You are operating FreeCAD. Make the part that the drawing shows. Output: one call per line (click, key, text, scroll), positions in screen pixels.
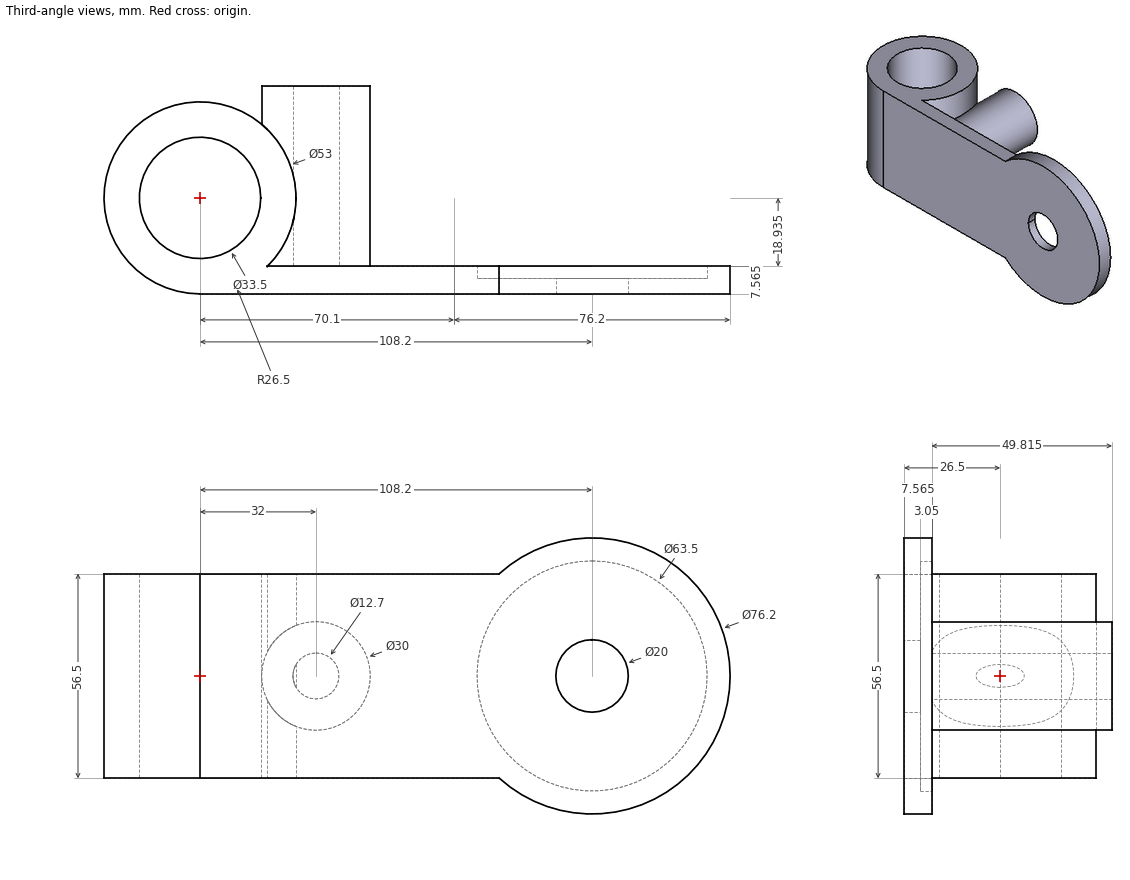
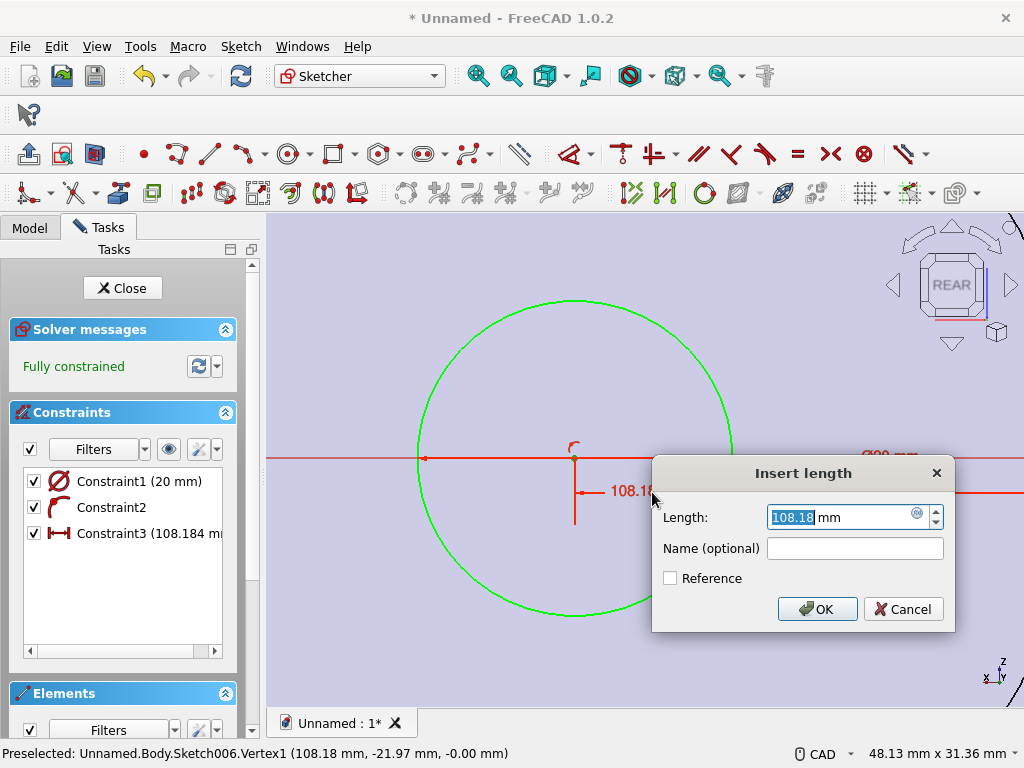
text(108.2)
key(Return)
key(Escape)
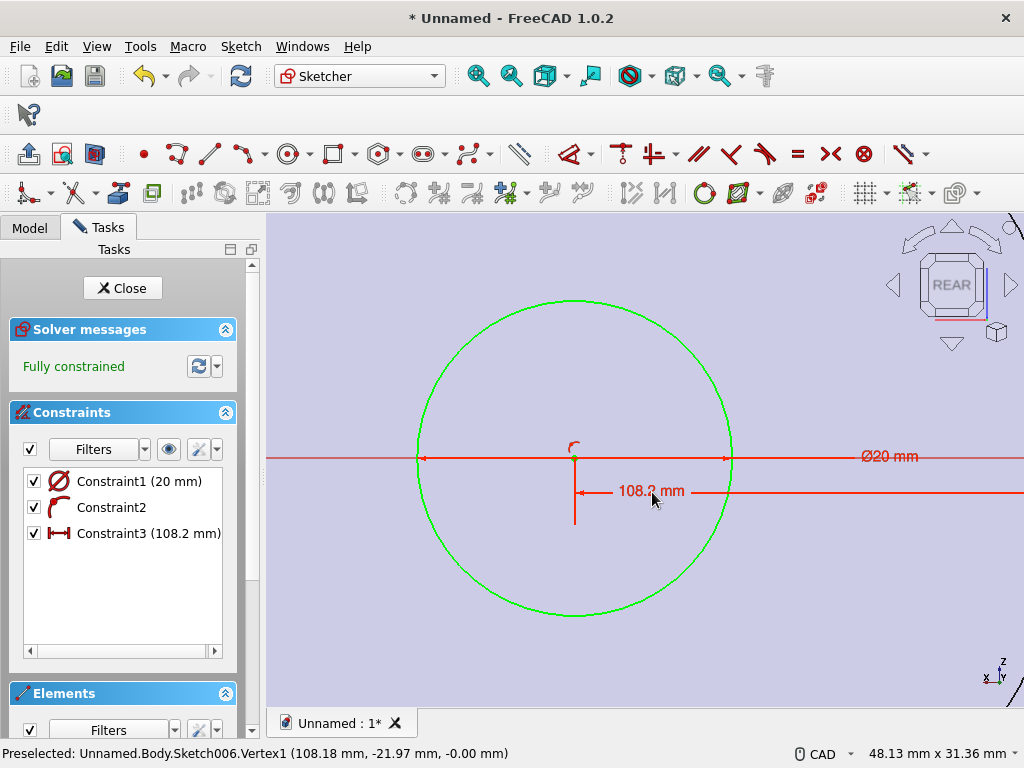
click(123, 288)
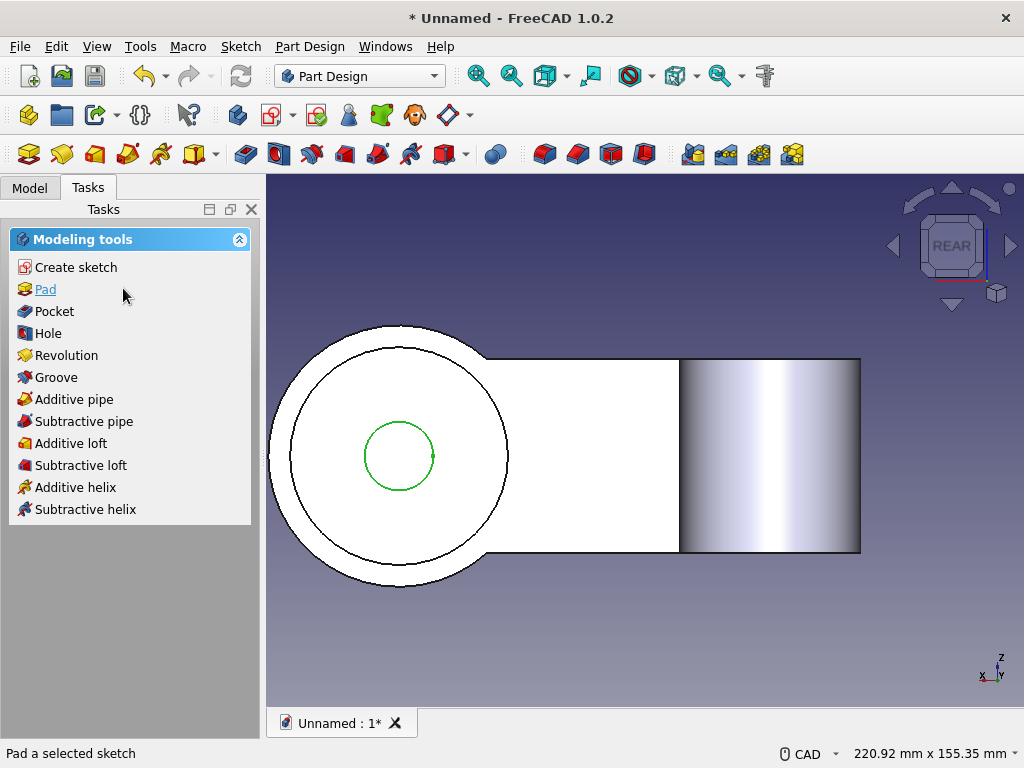
click(246, 154)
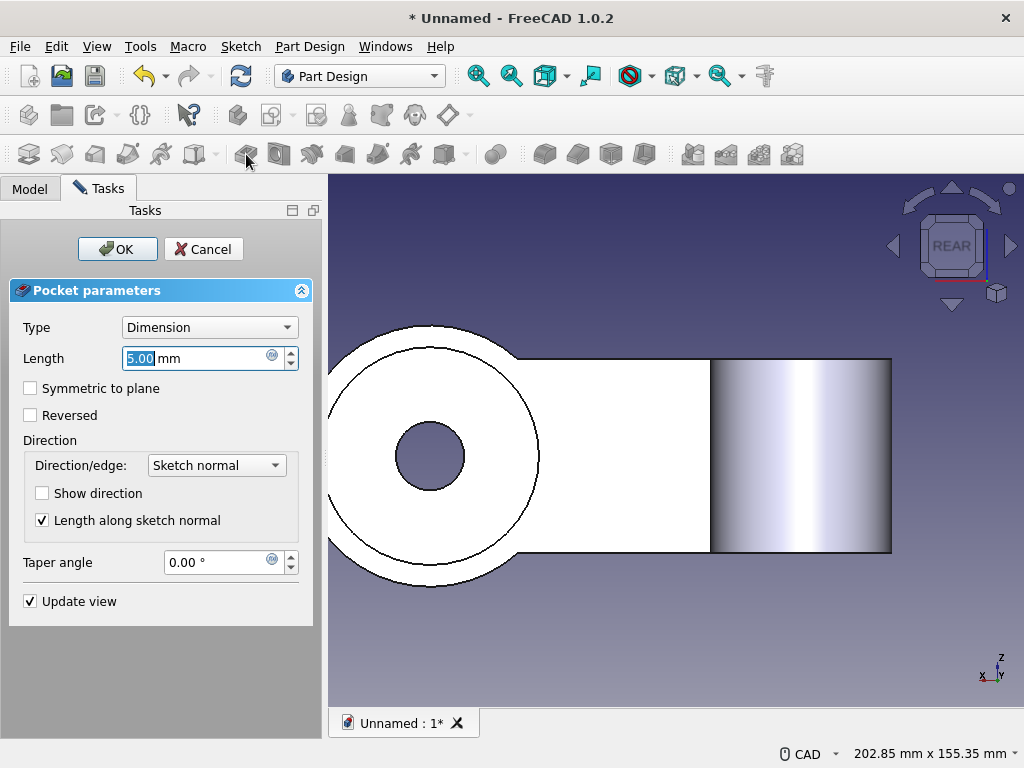
click(210, 328)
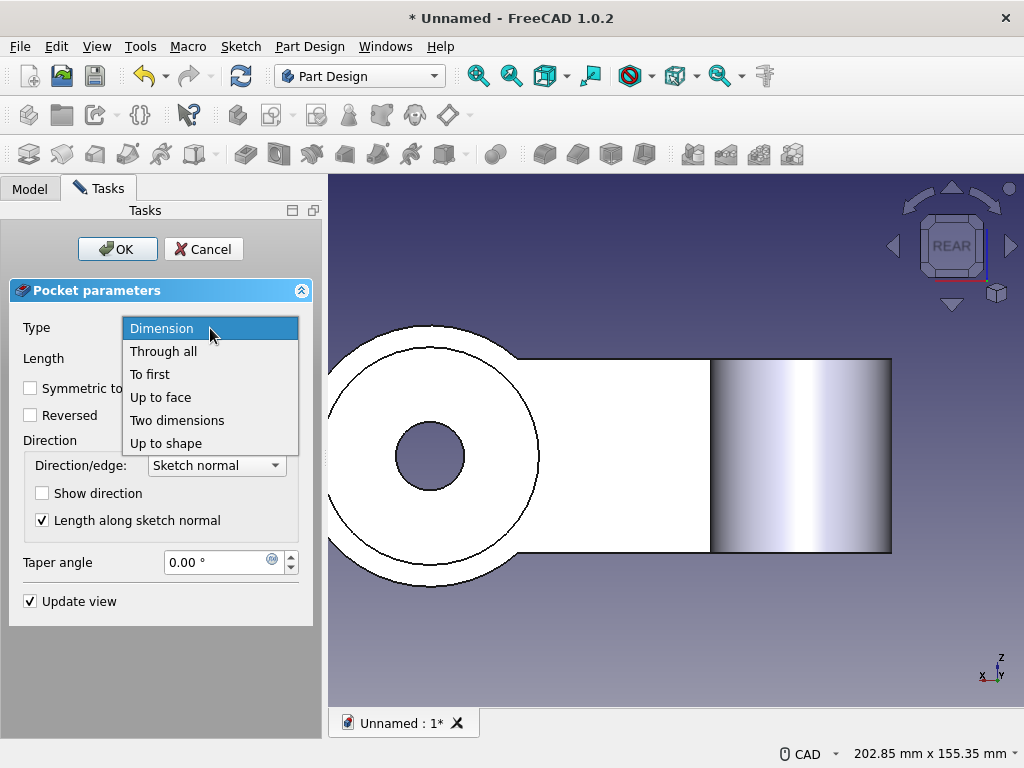
click(208, 352)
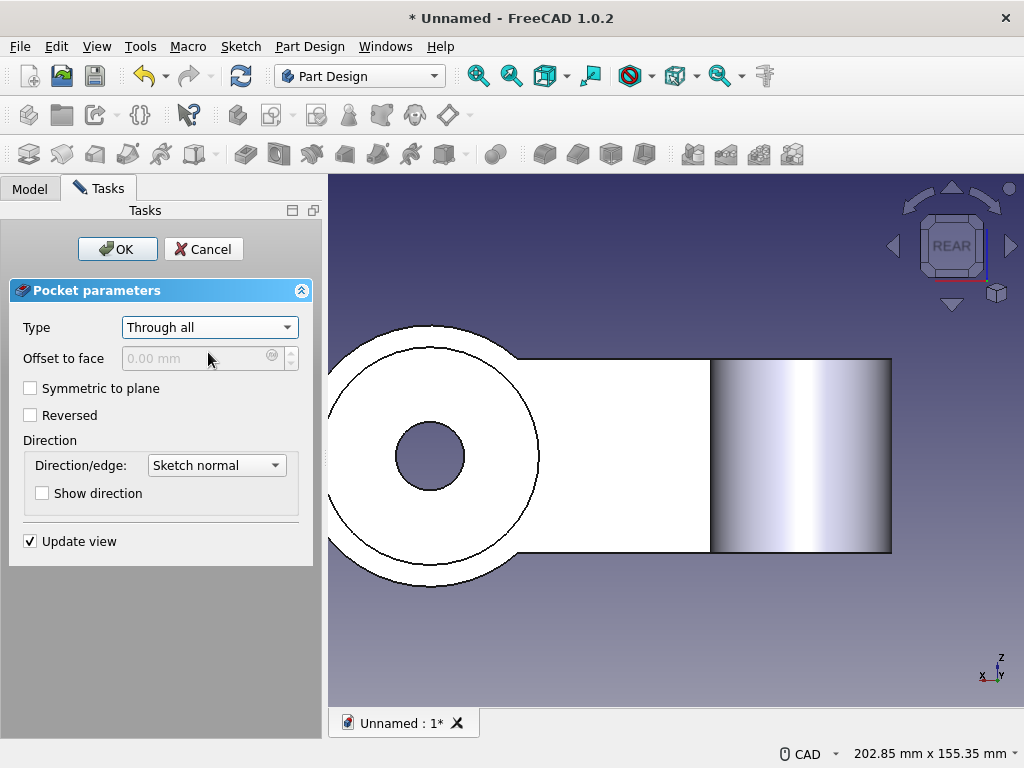
click(118, 249)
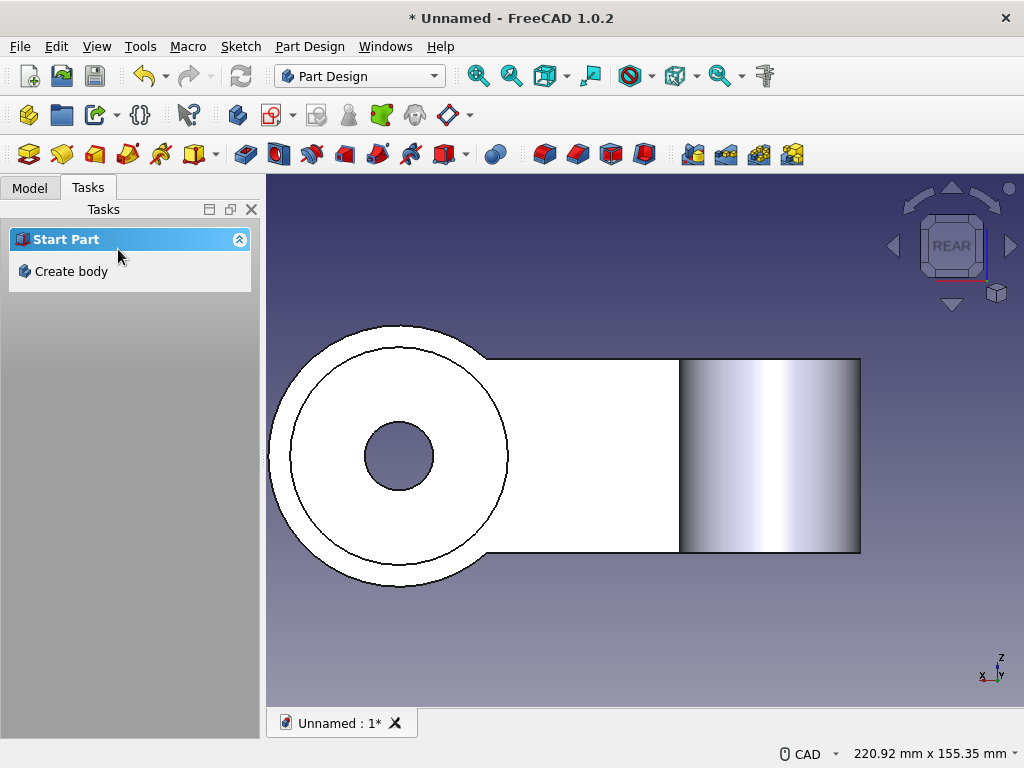
click(613, 455)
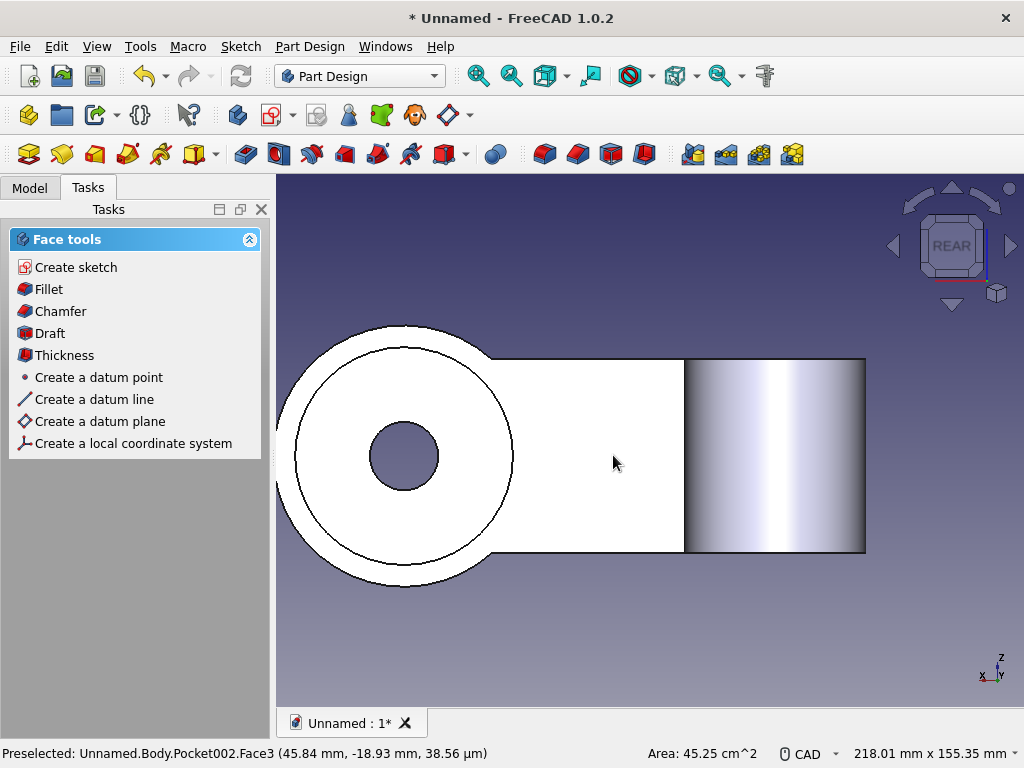
click(270, 116)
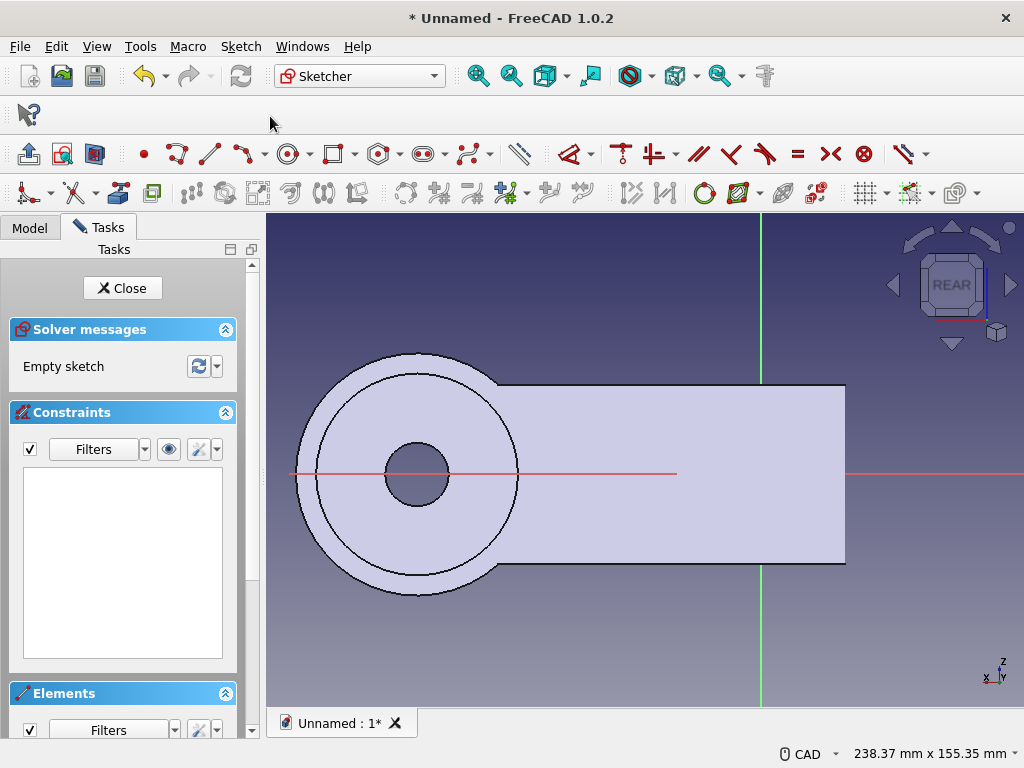
click(95, 154)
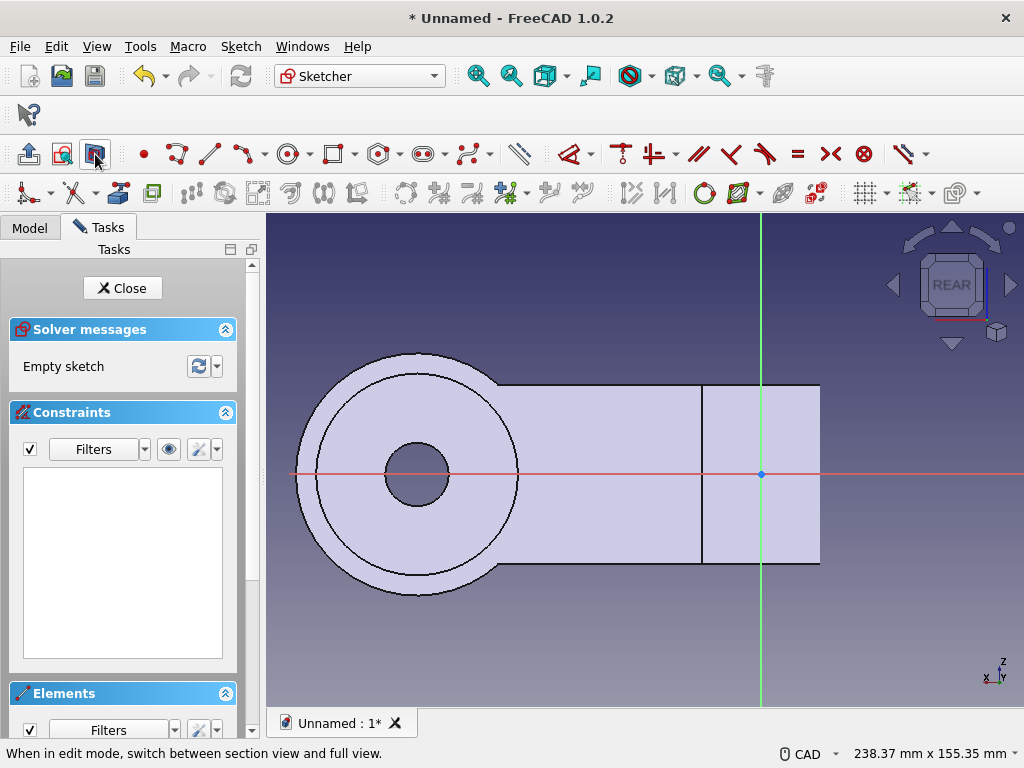
scroll(750, 483, up, 5)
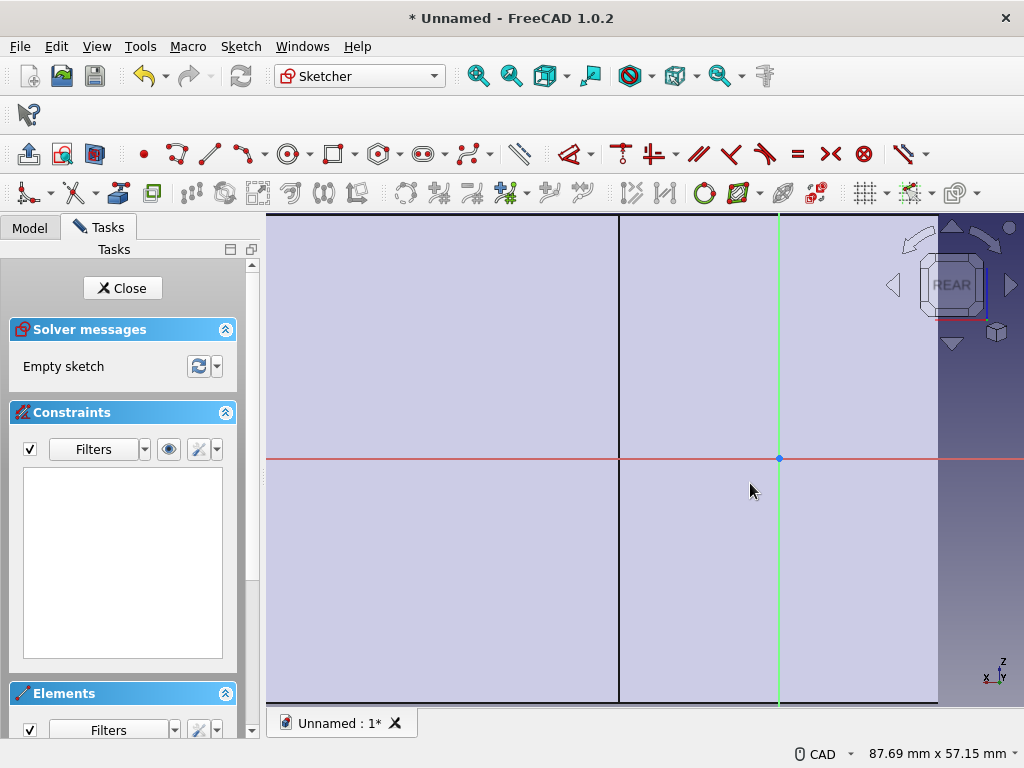
key(g)
key(c)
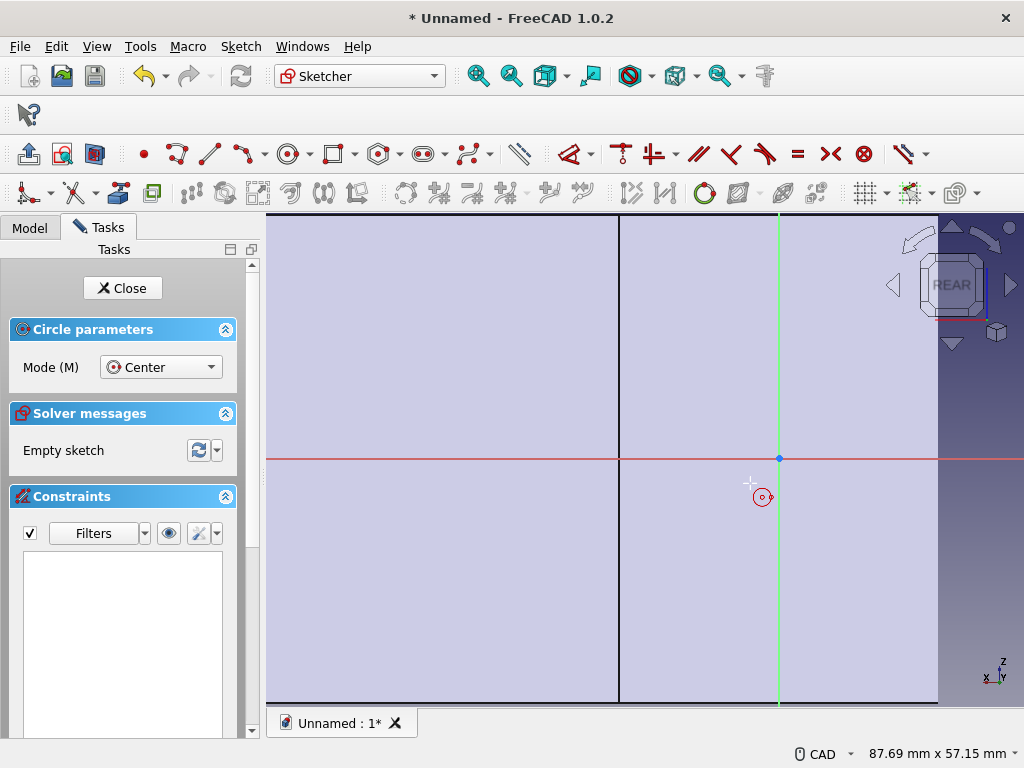
click(503, 459)
move(594, 367)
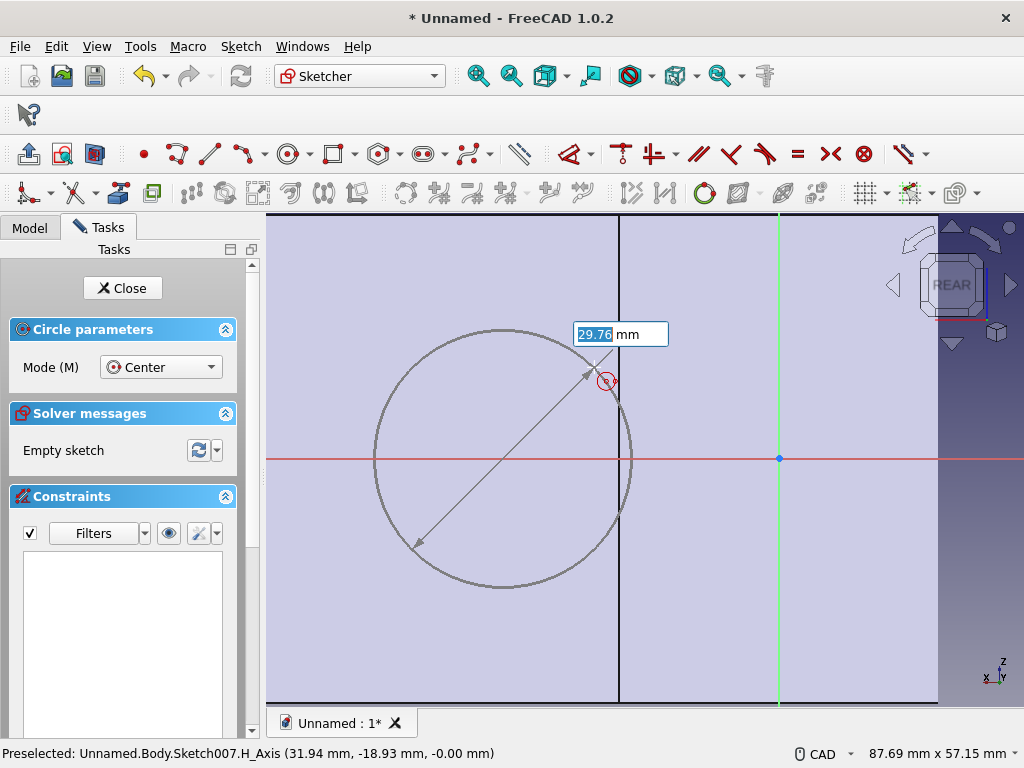
text(30)
key(Return)